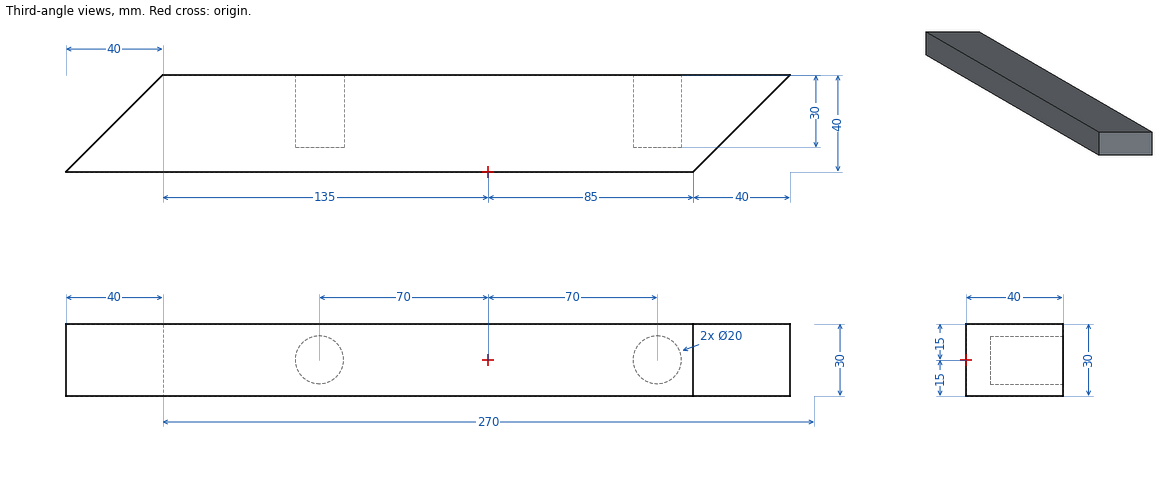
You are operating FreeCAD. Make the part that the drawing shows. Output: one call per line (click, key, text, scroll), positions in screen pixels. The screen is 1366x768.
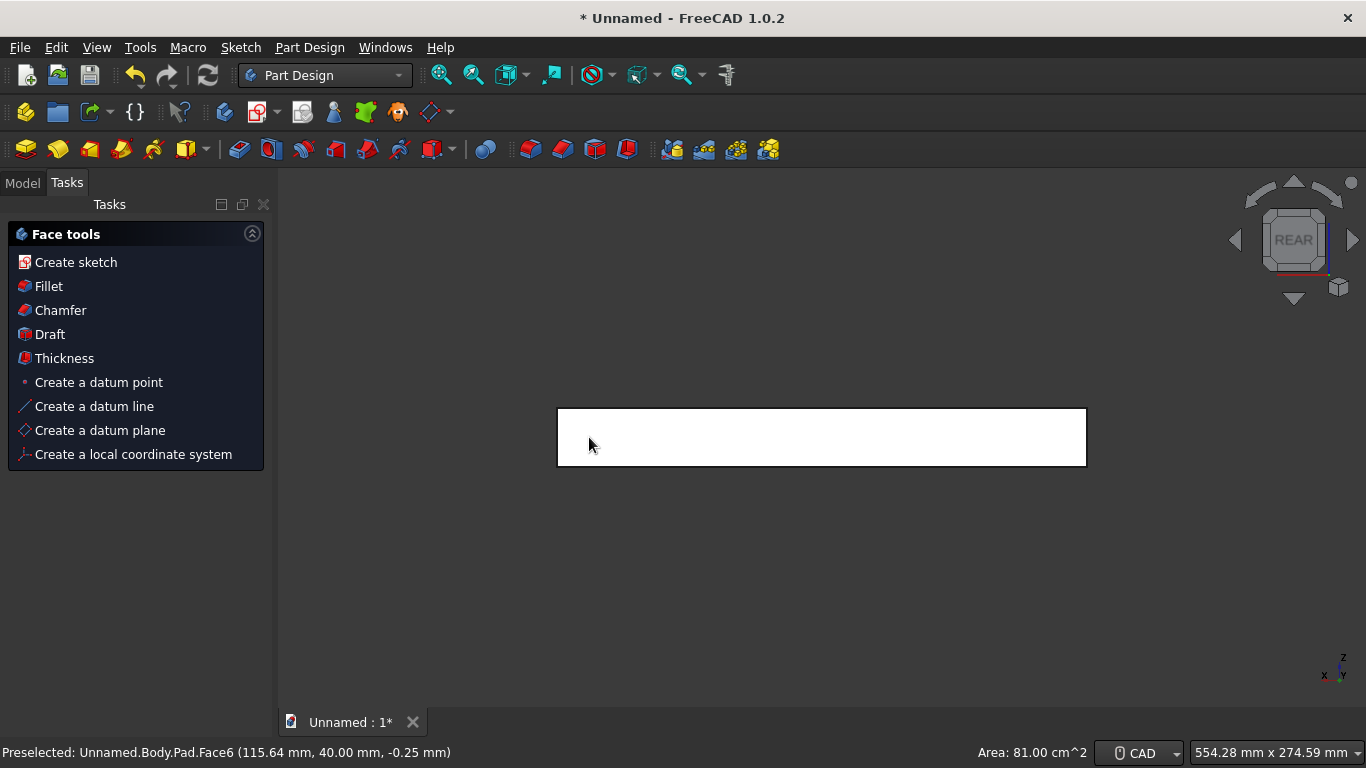
click(258, 112)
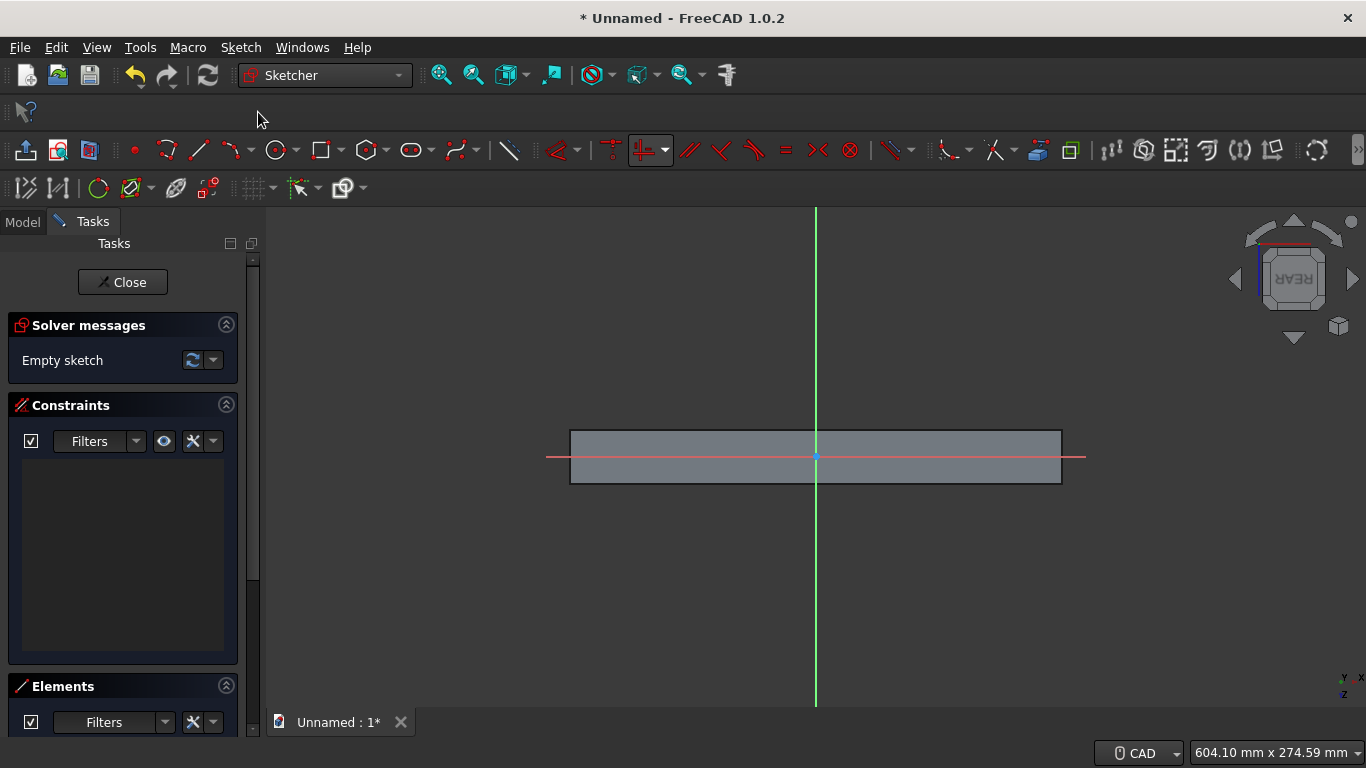
scroll(872, 457, up, 4)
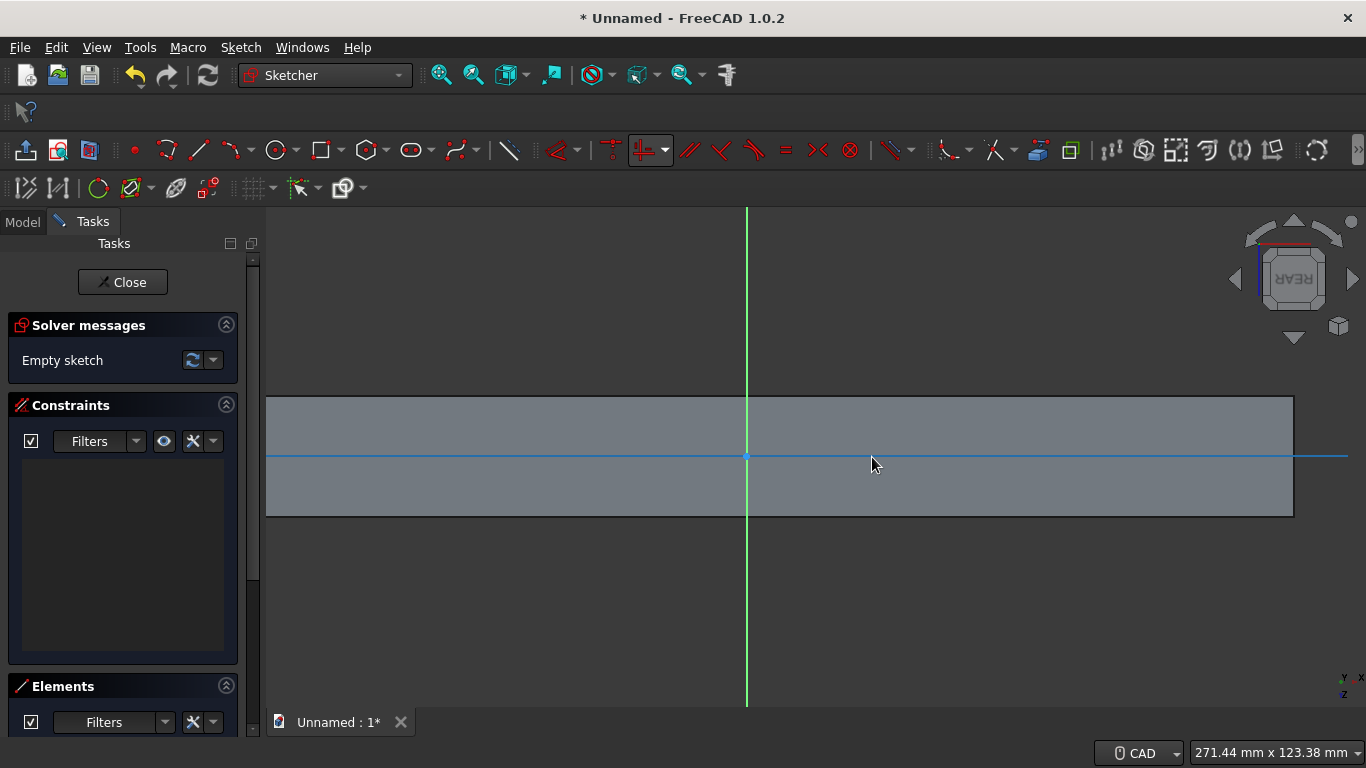
click(276, 150)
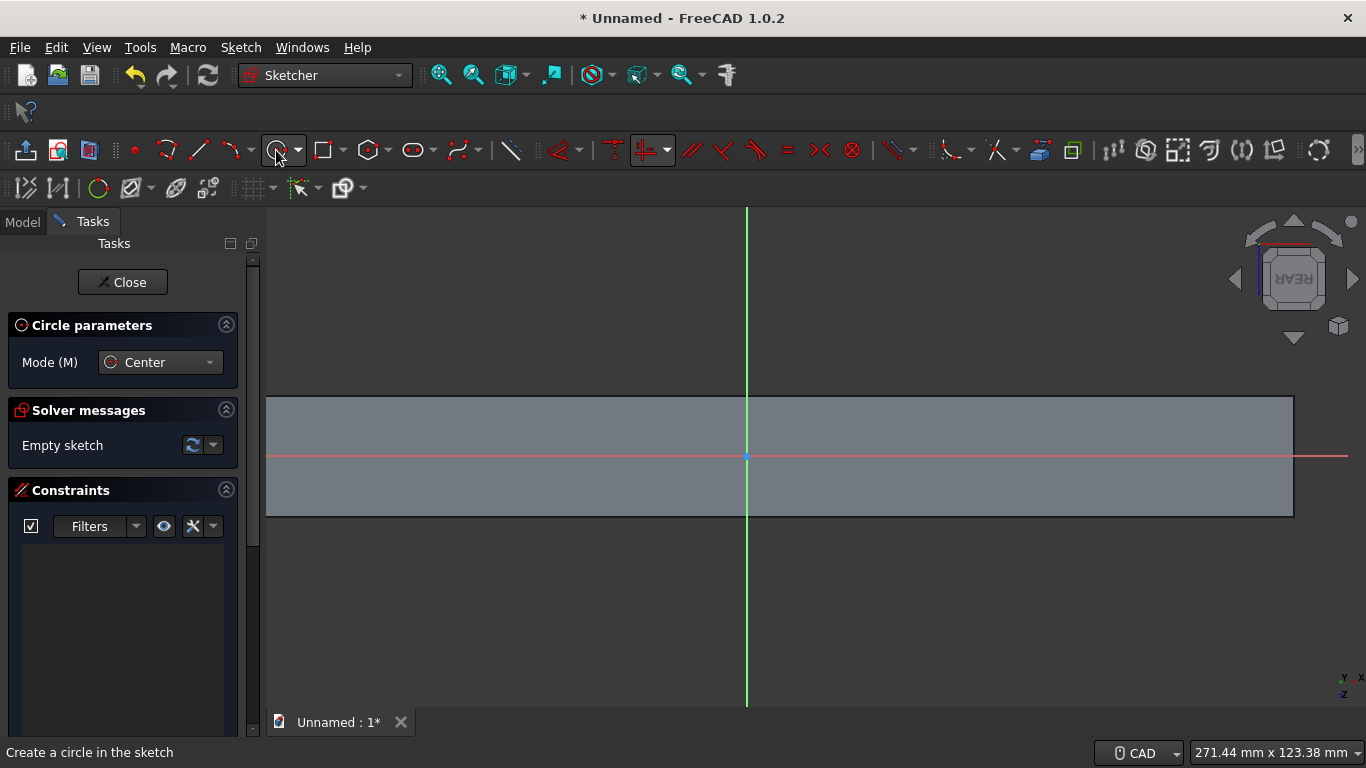
click(1030, 456)
click(1059, 428)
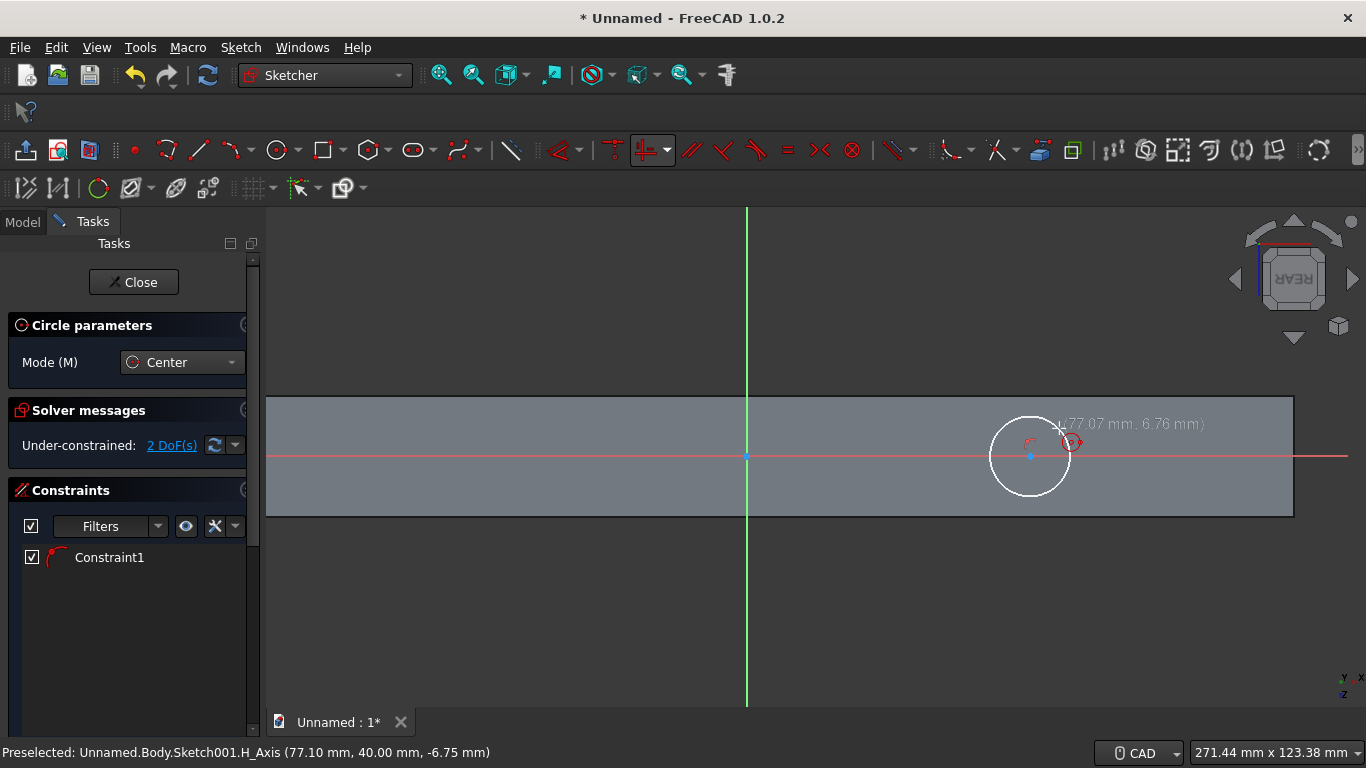
click(463, 456)
click(492, 428)
key(Escape)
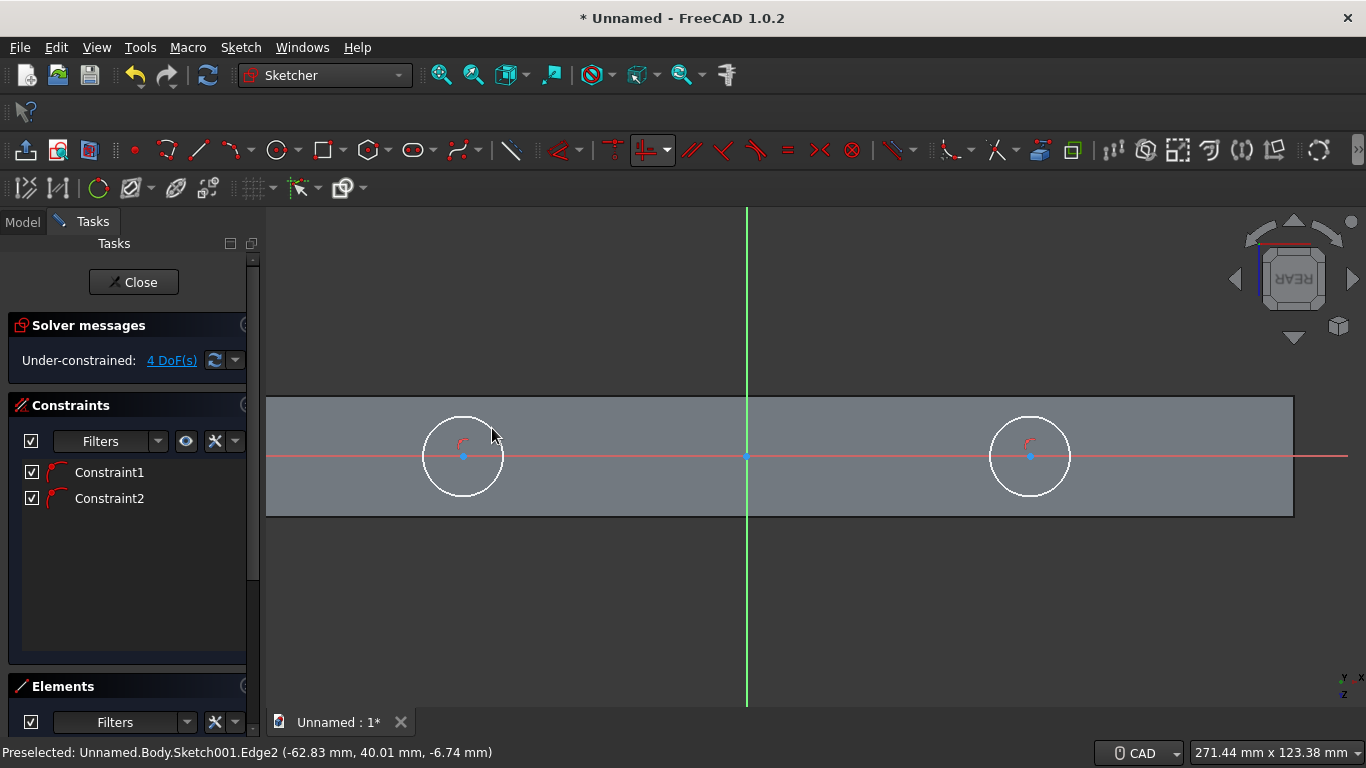
click(1058, 428)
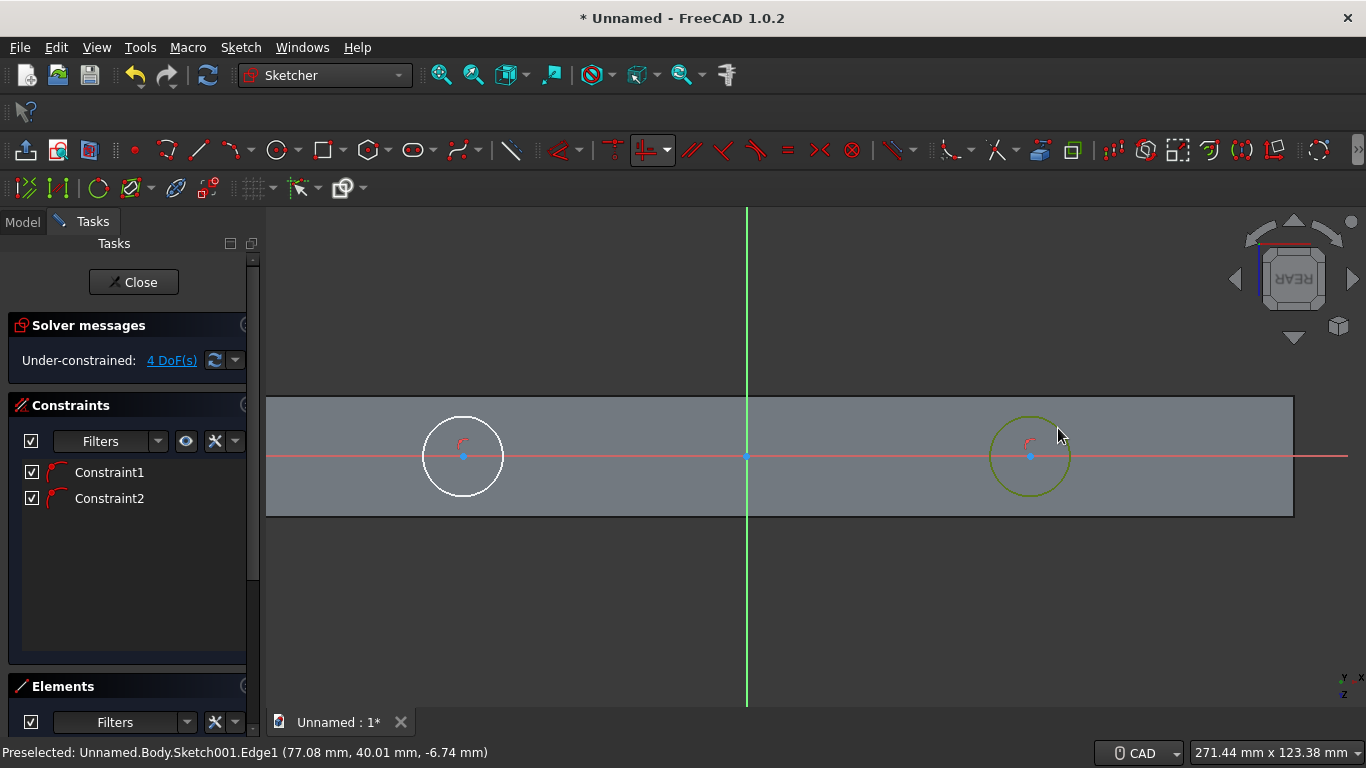
click(491, 428)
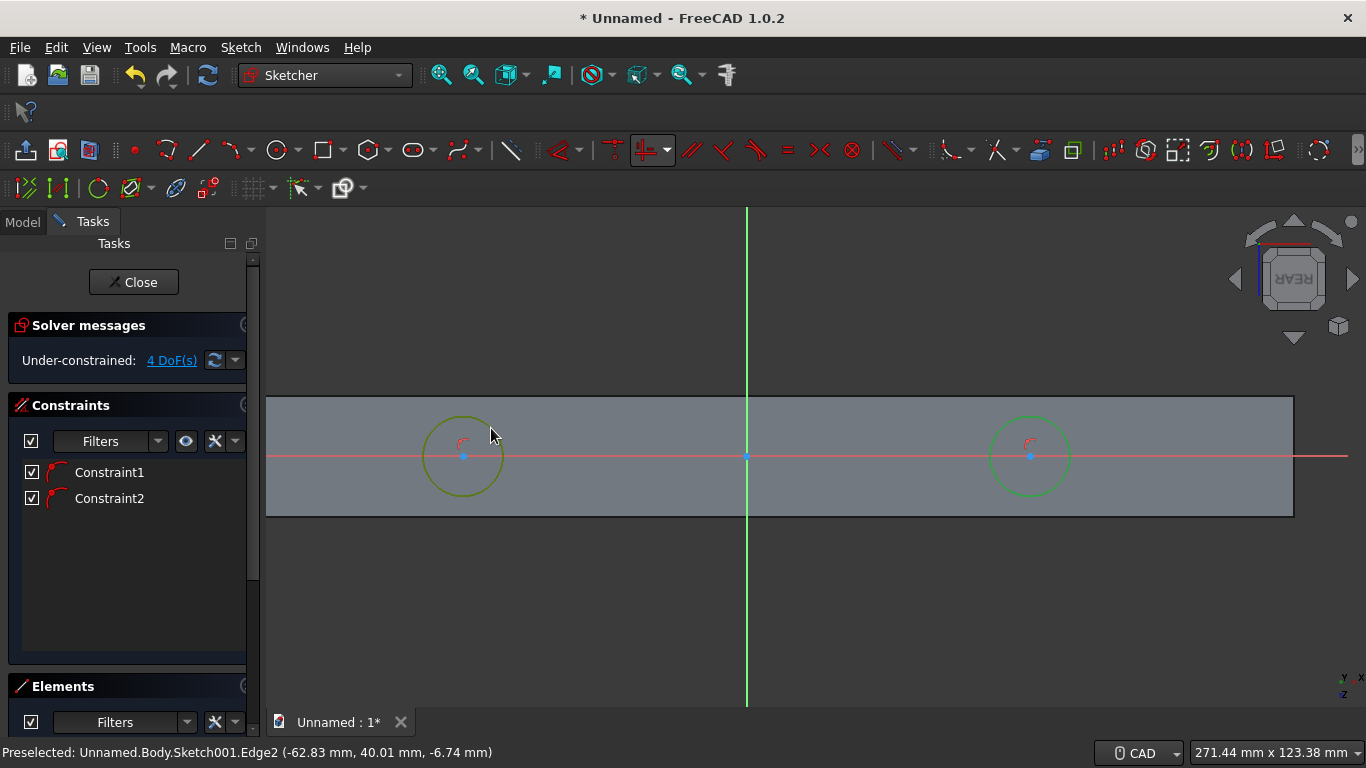
click(788, 150)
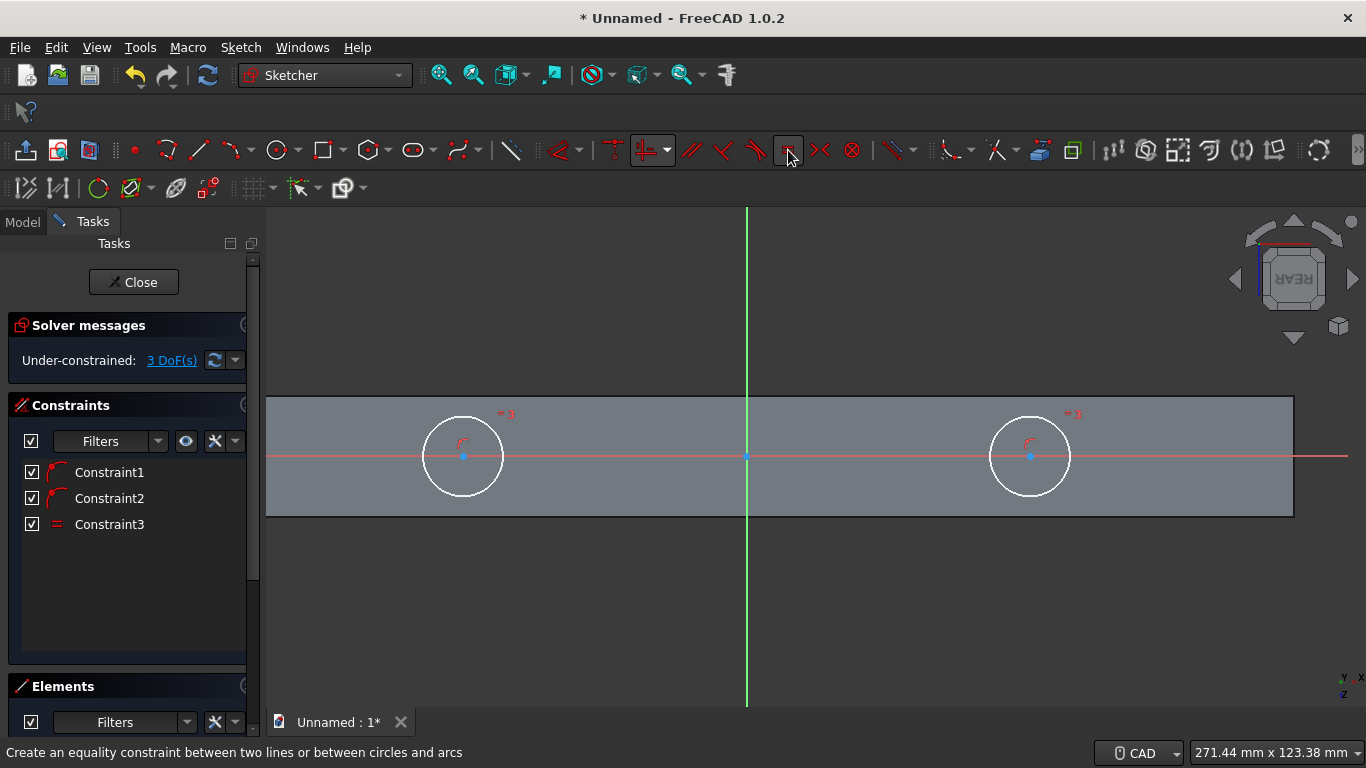
click(558, 150)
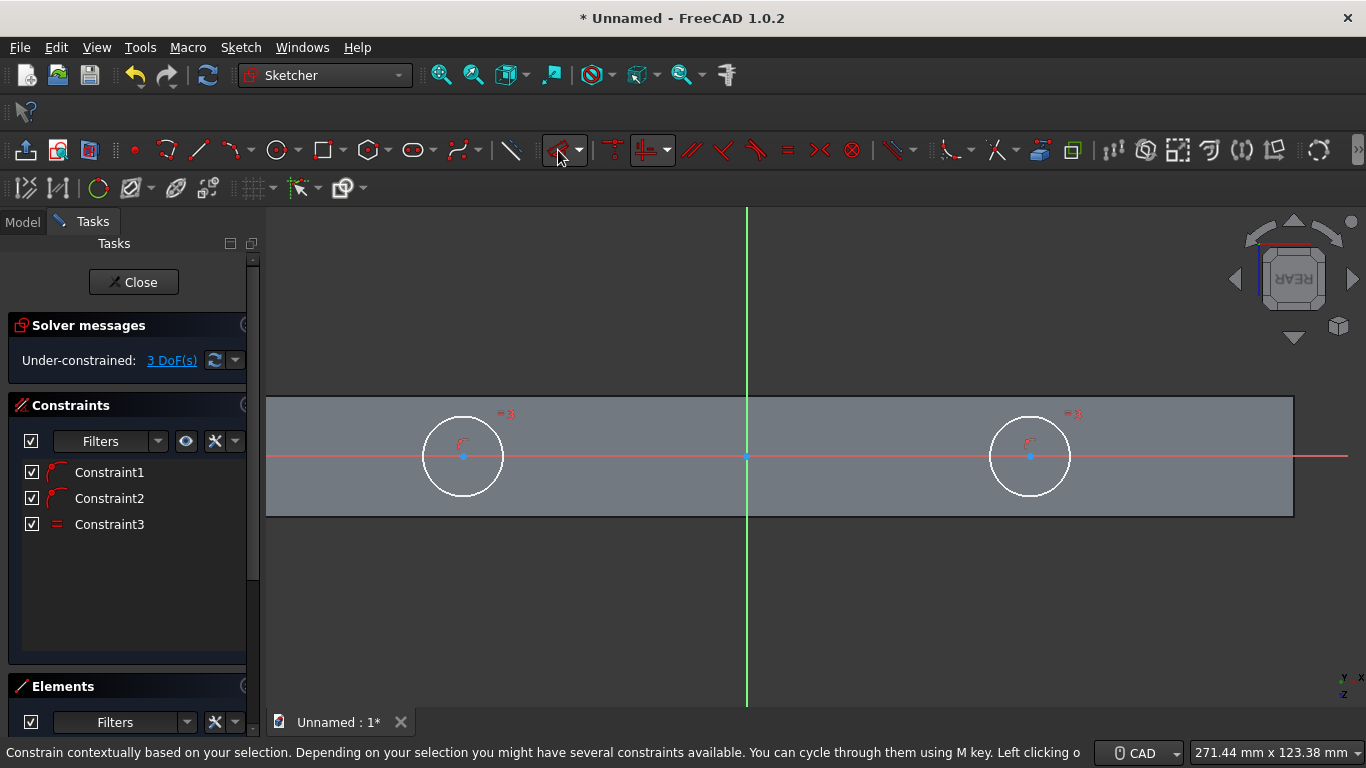
click(1058, 428)
click(1080, 405)